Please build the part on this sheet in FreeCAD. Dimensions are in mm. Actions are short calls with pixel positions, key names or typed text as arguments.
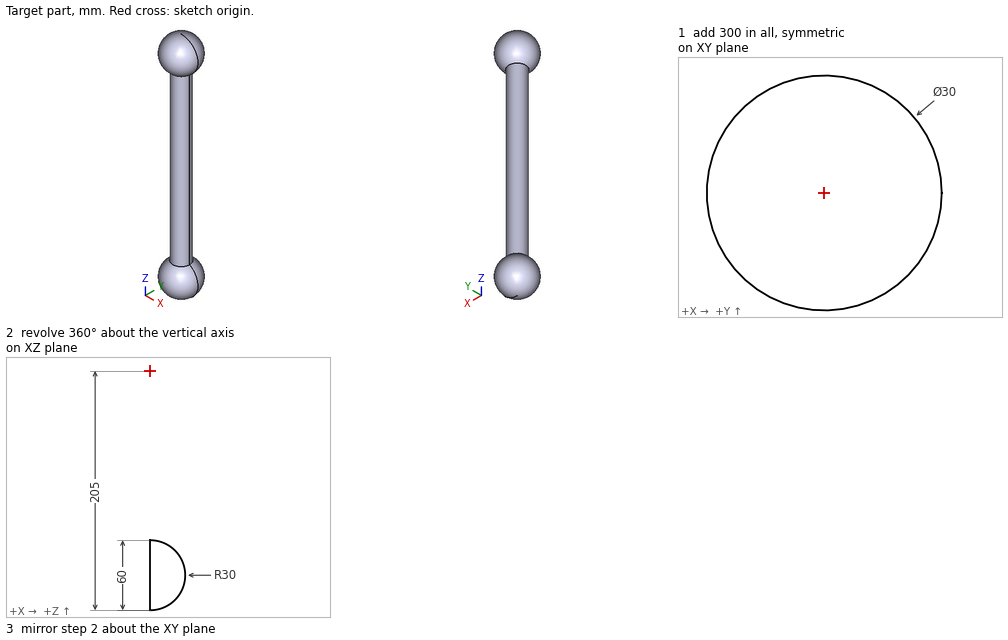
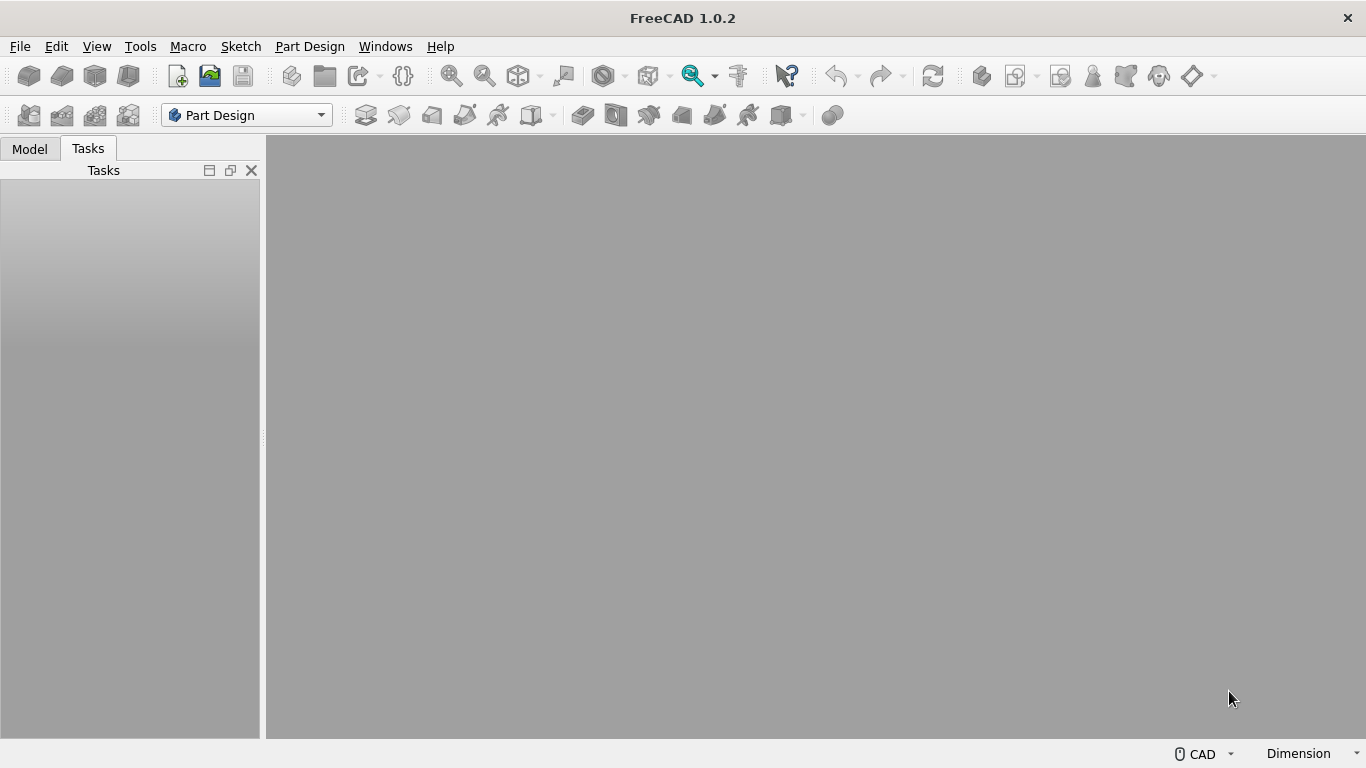
click(177, 76)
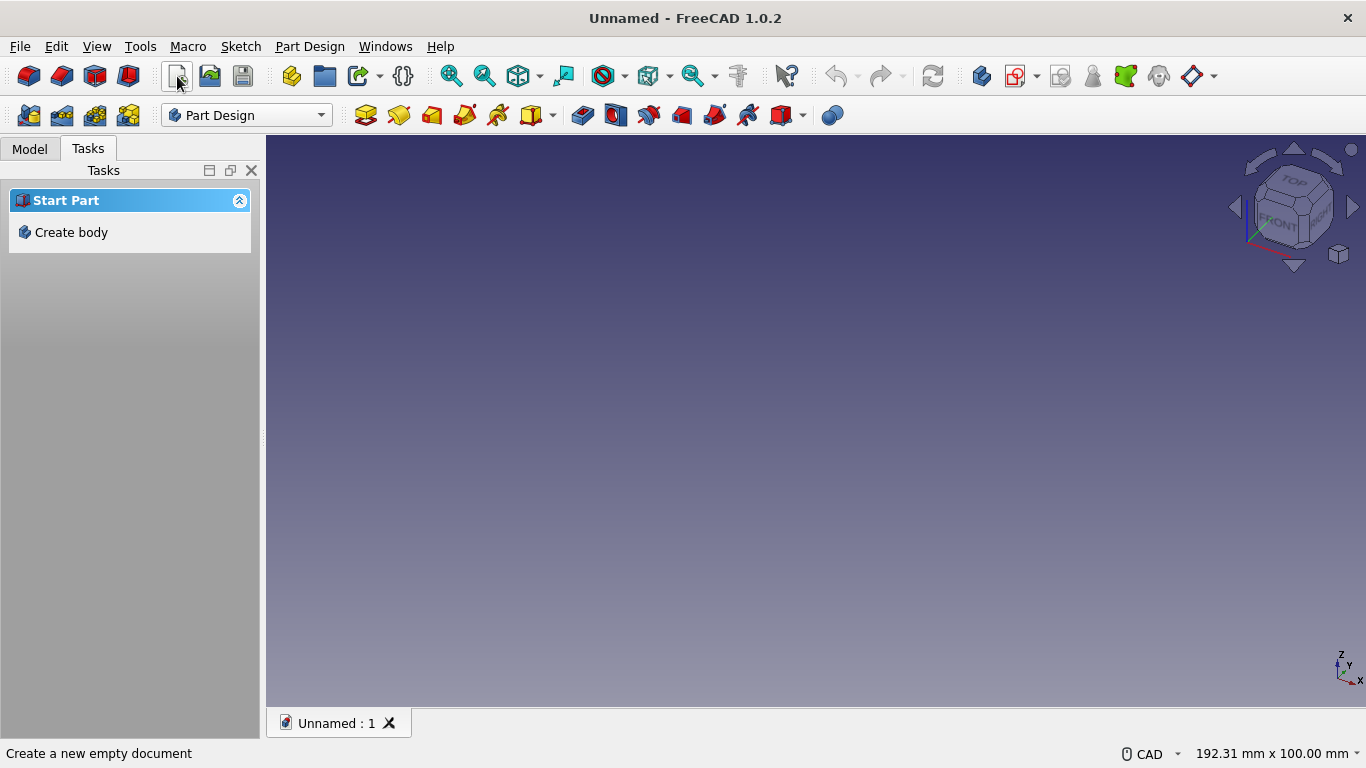
click(1014, 76)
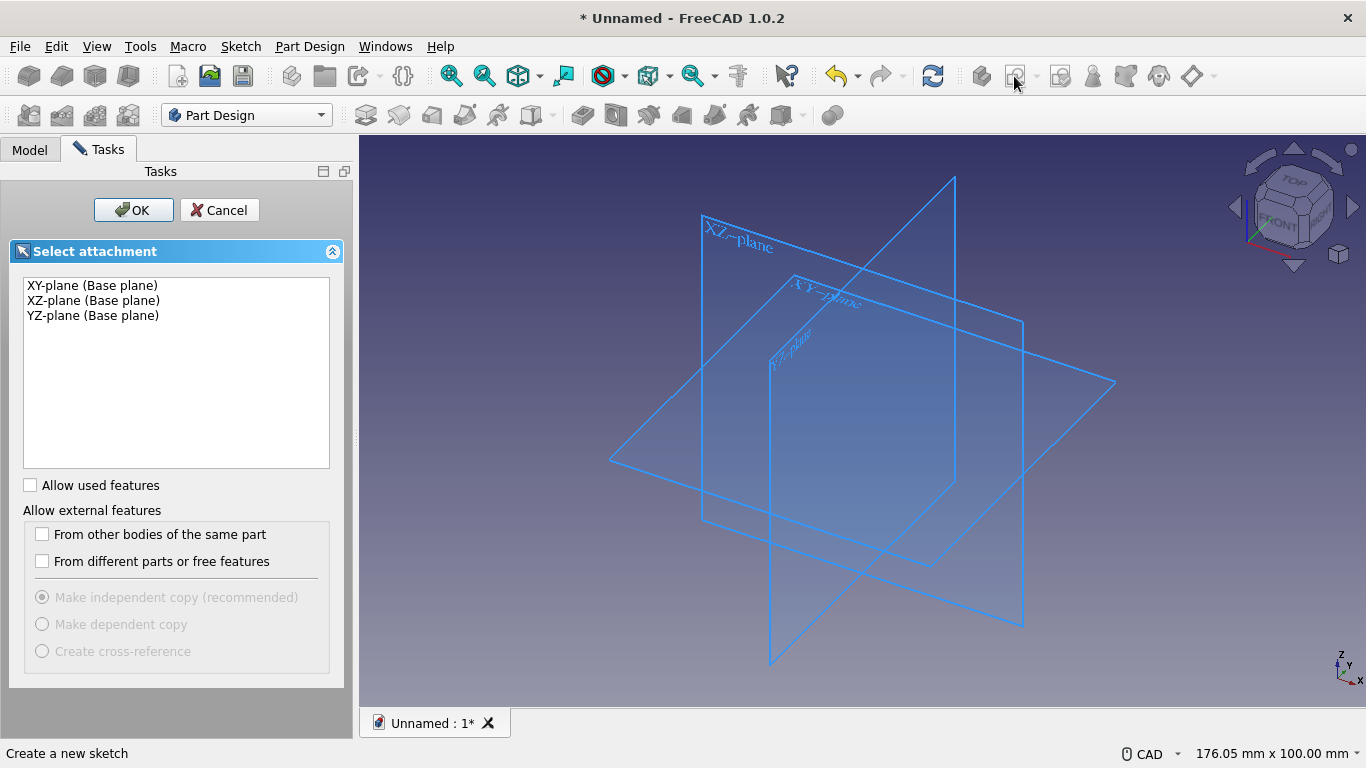
click(84, 286)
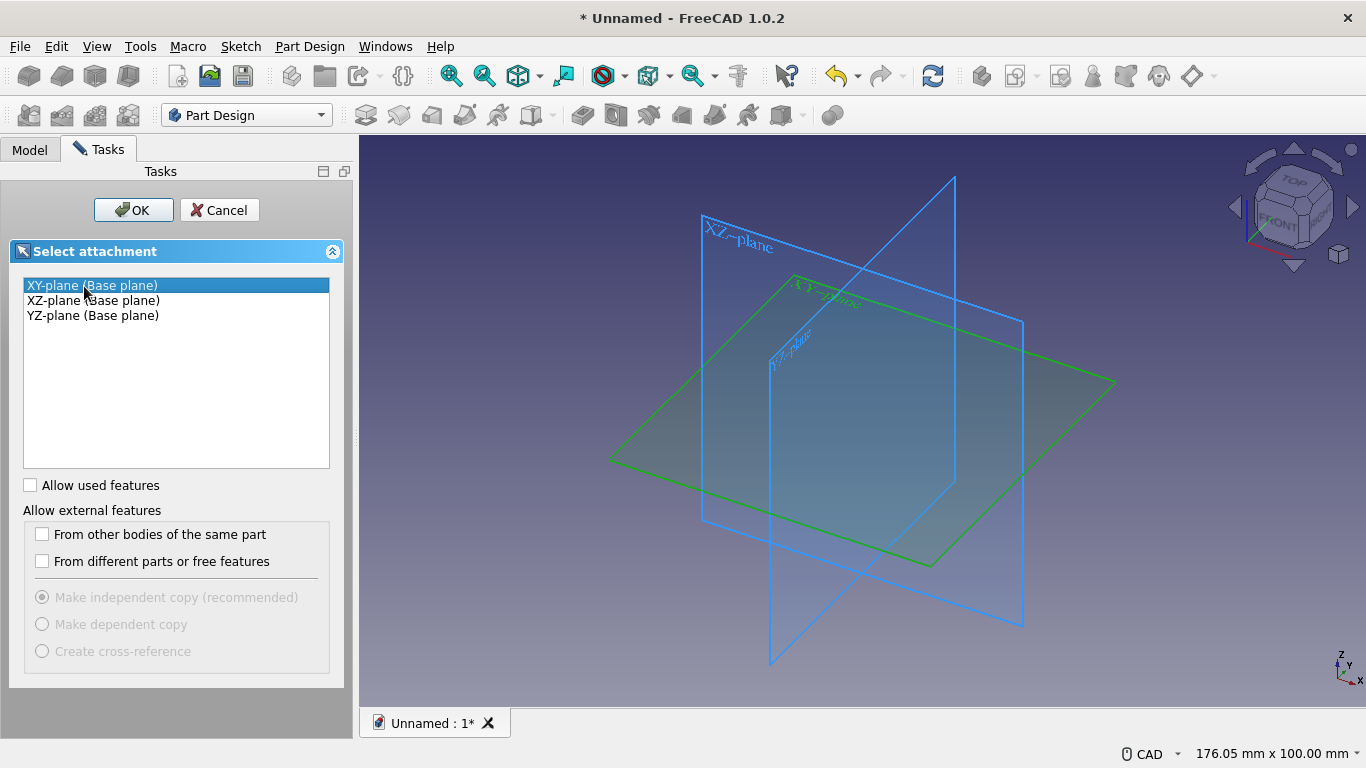
click(134, 210)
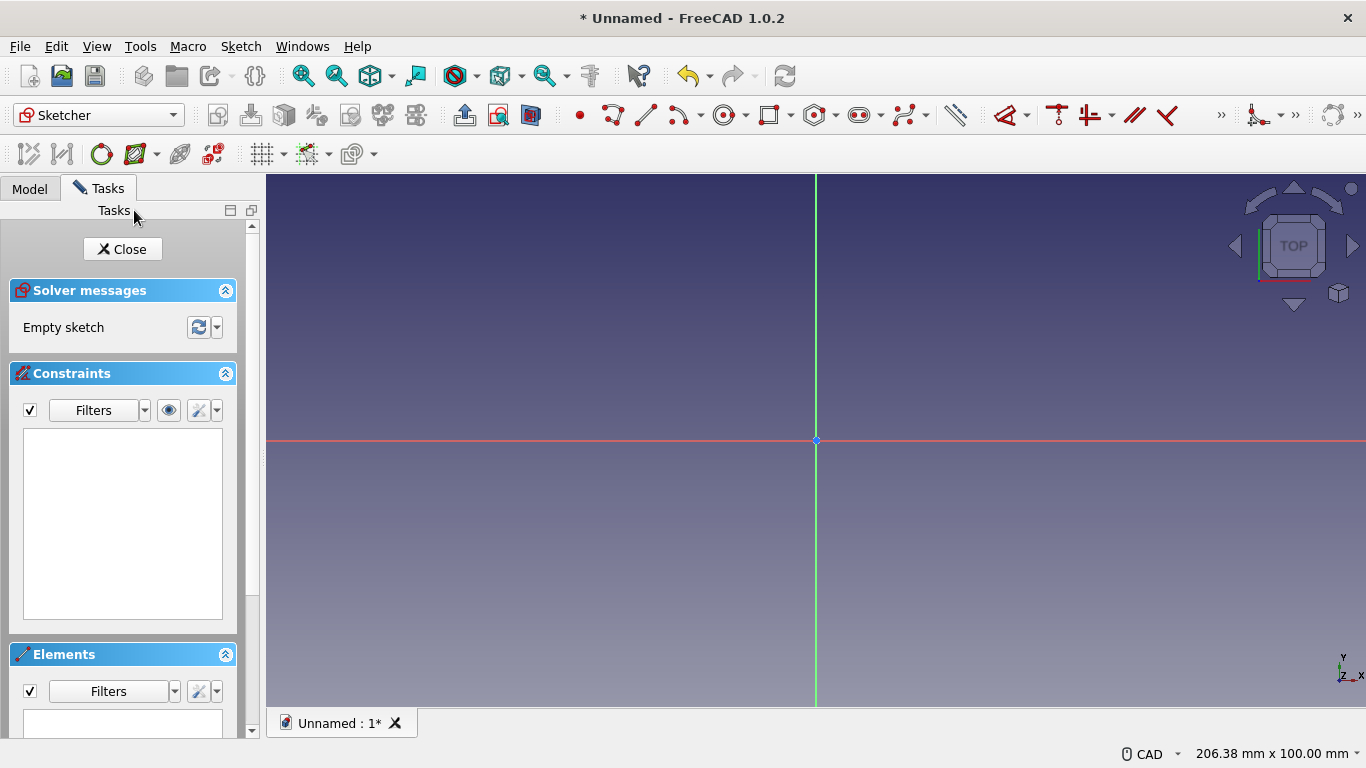
scroll(872, 440, up, 4)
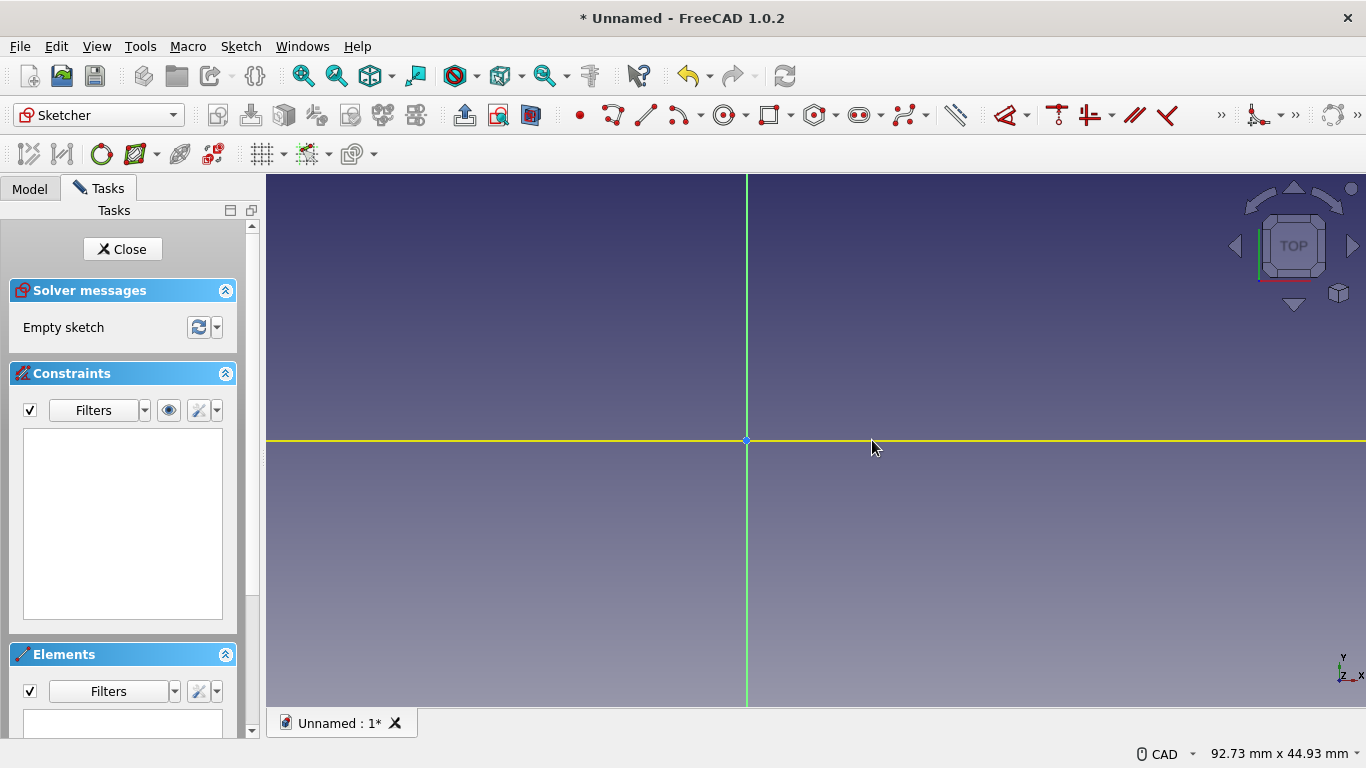
click(724, 116)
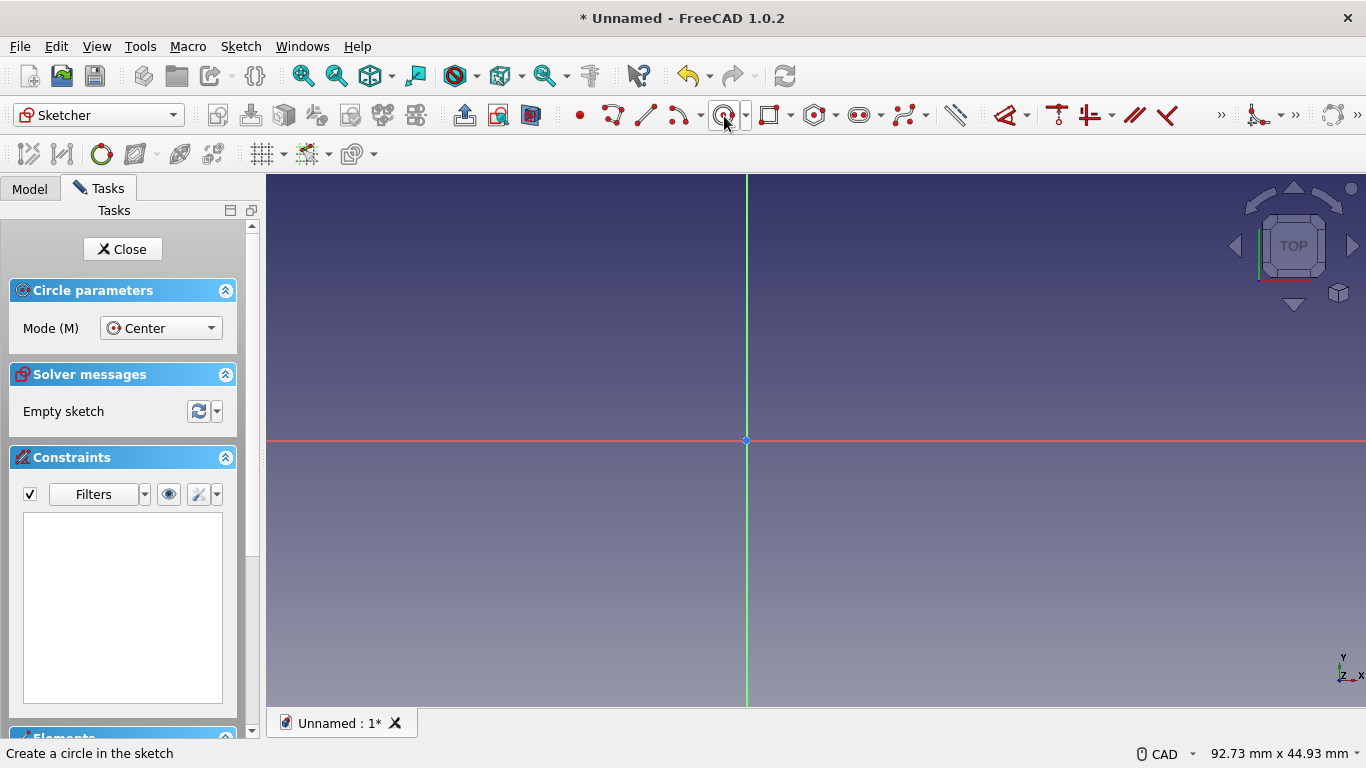
click(747, 440)
move(873, 315)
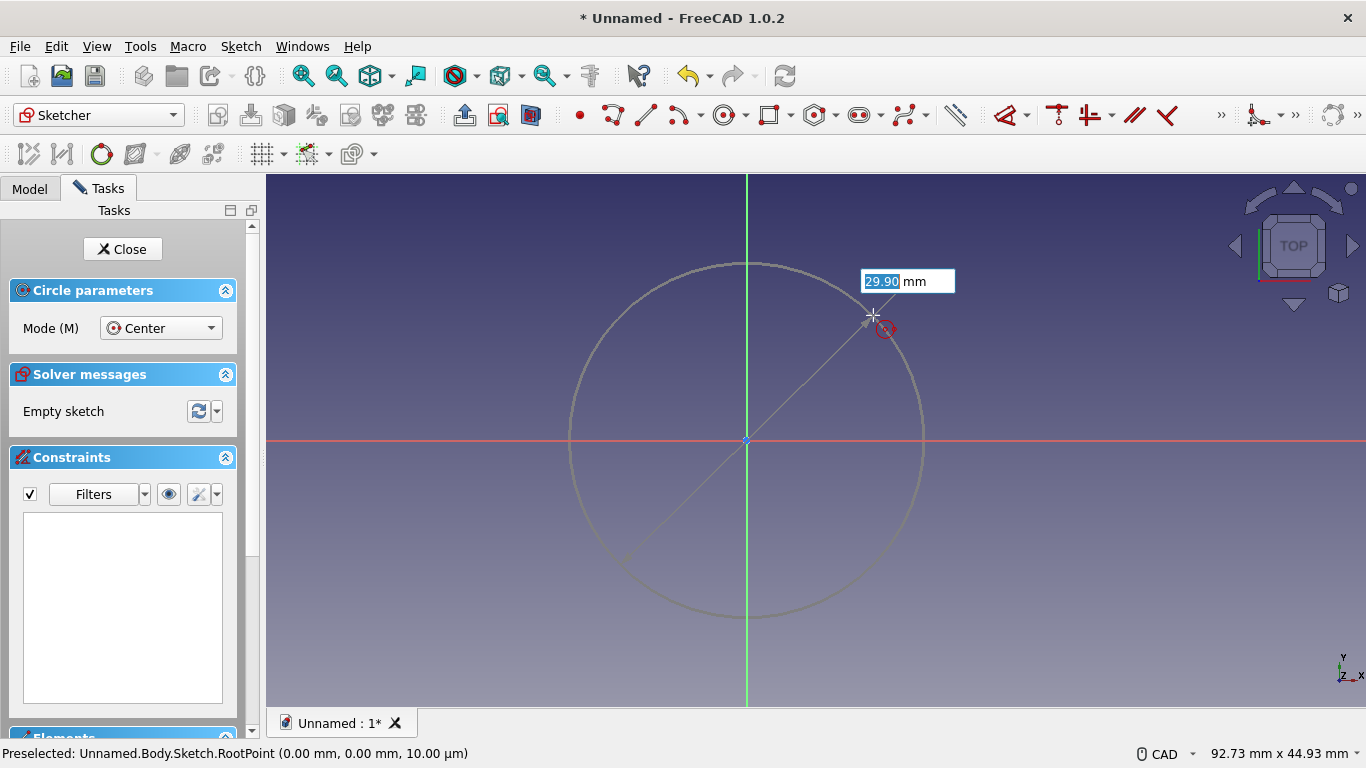
text(30)
key(Return)
key(Escape)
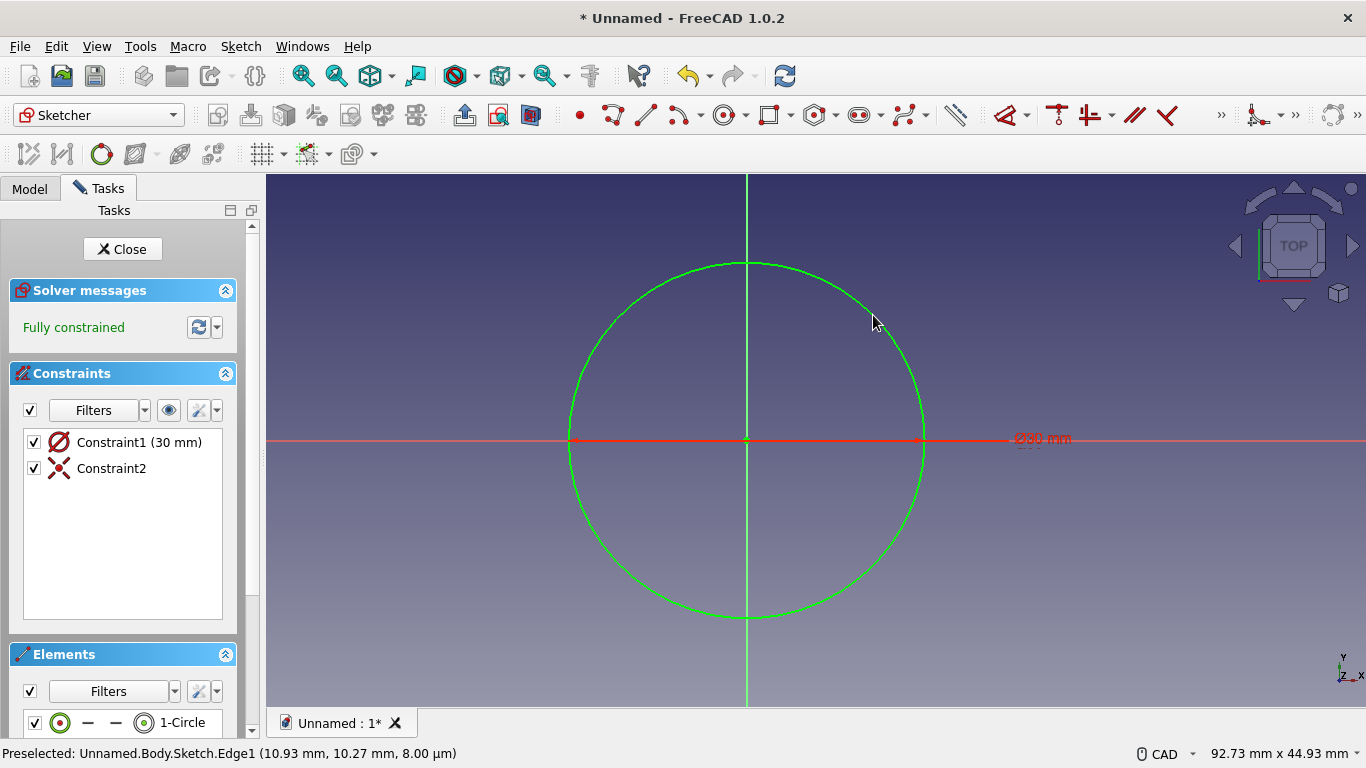
click(123, 249)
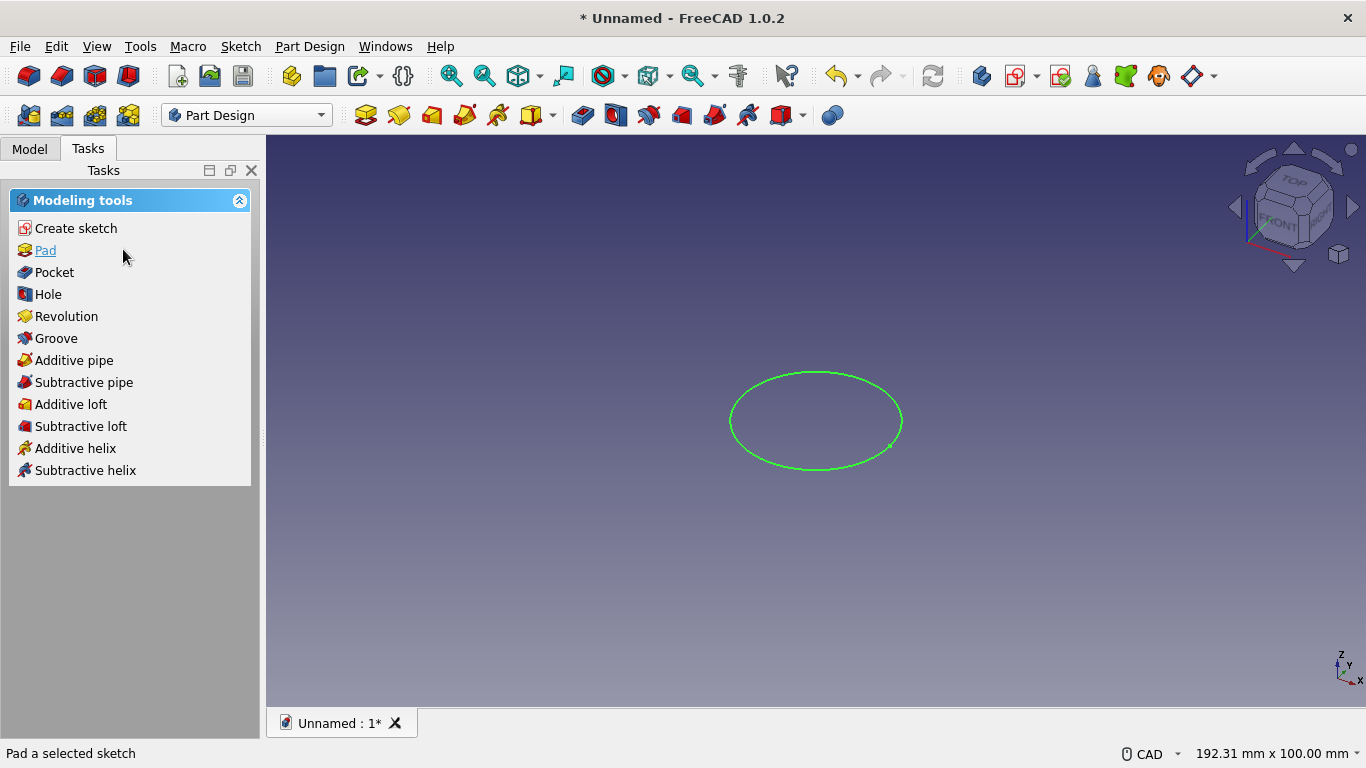
click(366, 116)